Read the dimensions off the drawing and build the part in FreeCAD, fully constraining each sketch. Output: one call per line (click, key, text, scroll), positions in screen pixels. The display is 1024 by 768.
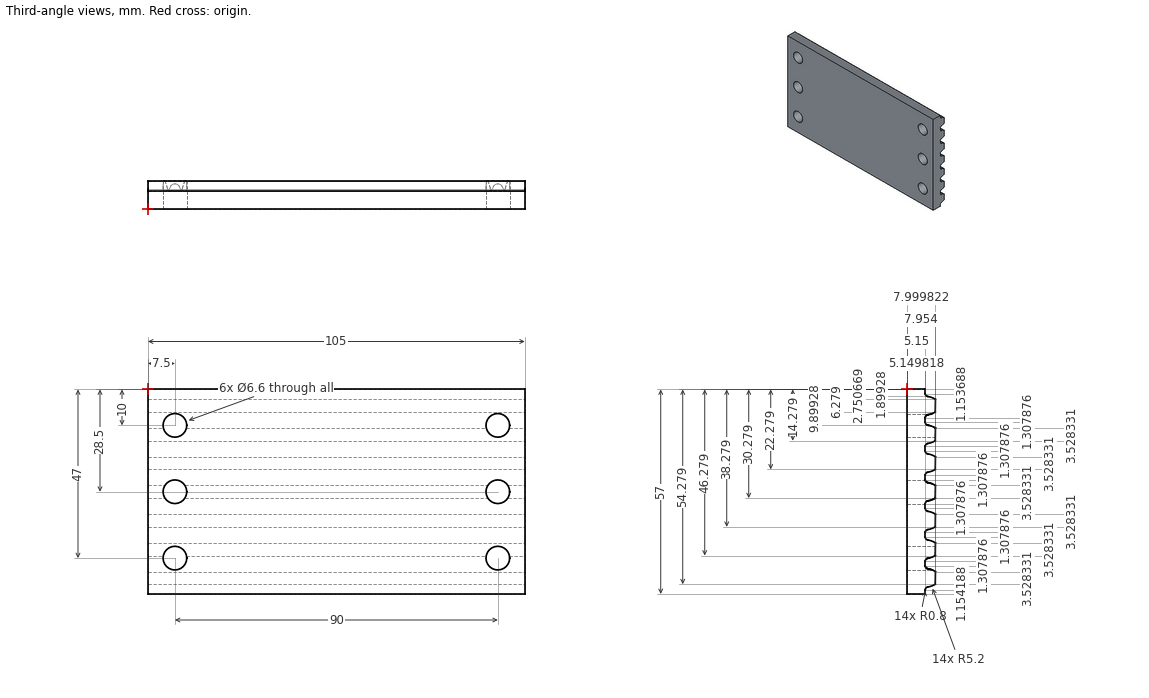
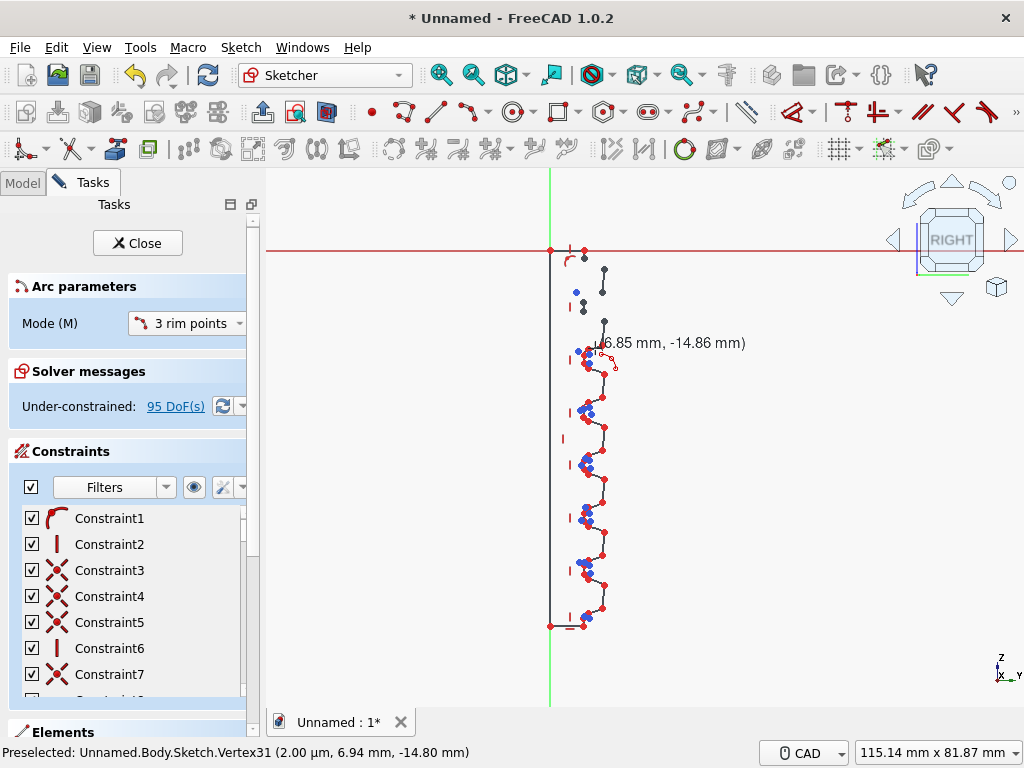
scroll(603, 321, up, 2)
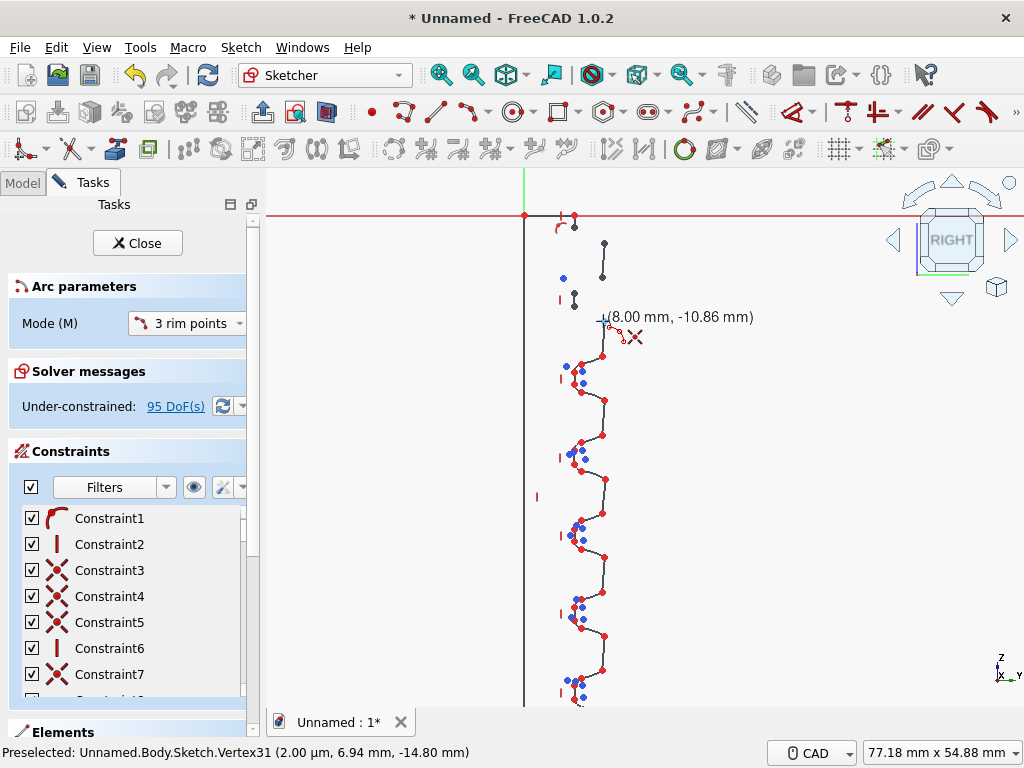
click(605, 322)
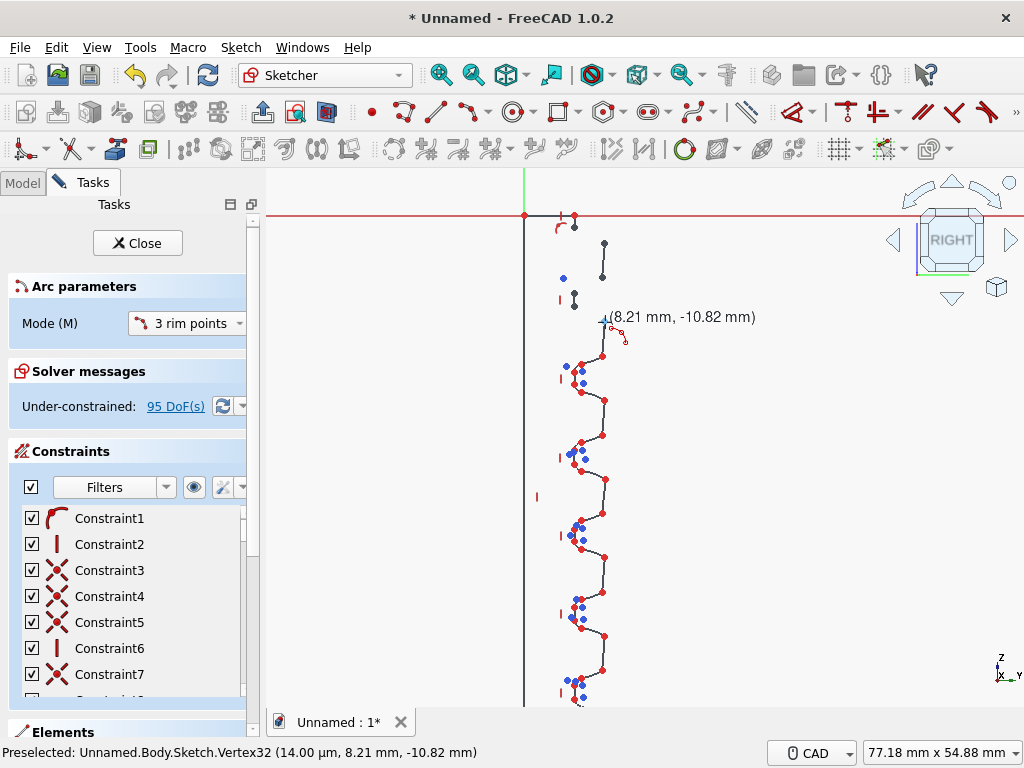
scroll(582, 313, up, 5)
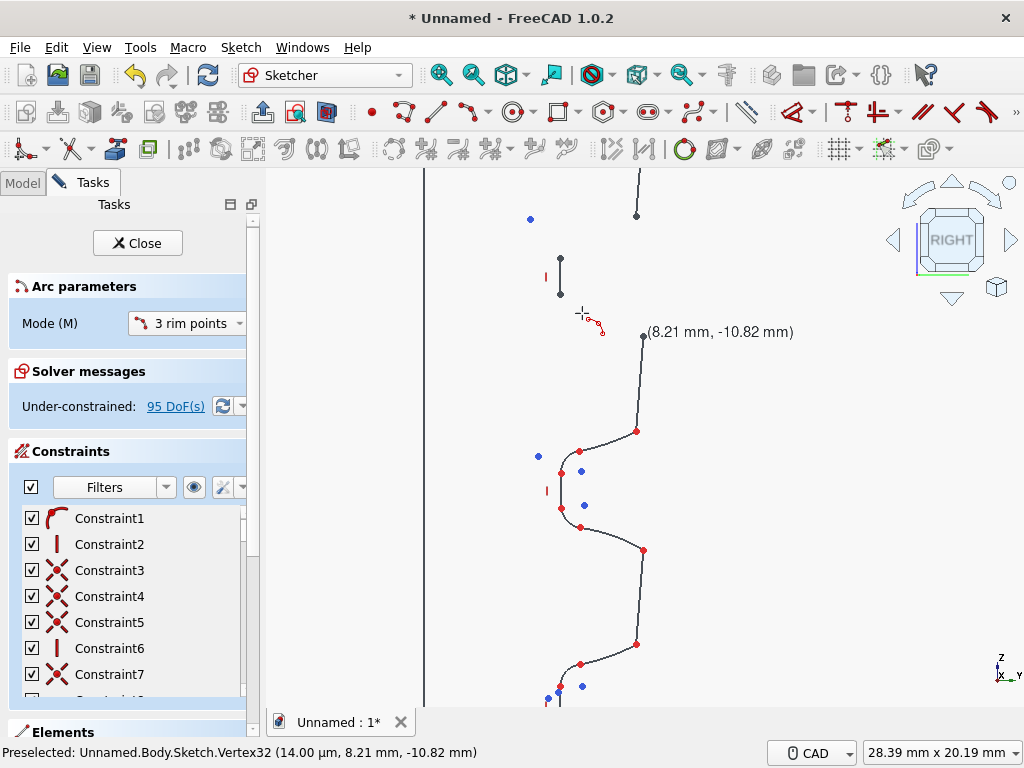
click(580, 314)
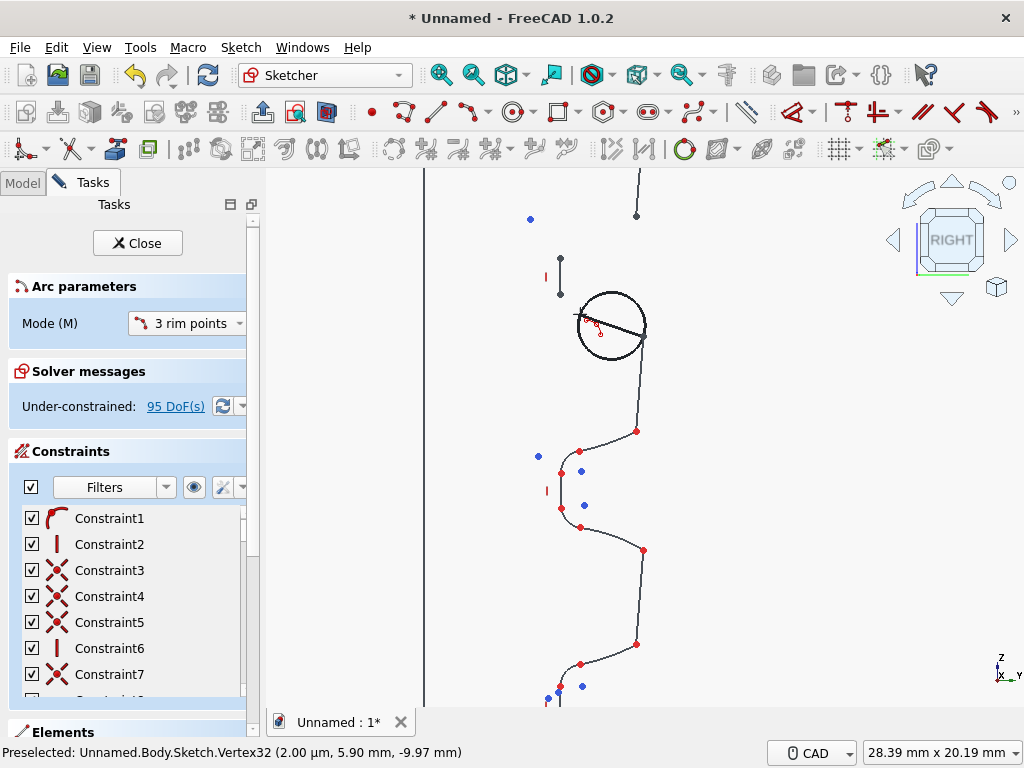
scroll(610, 321, up, 8)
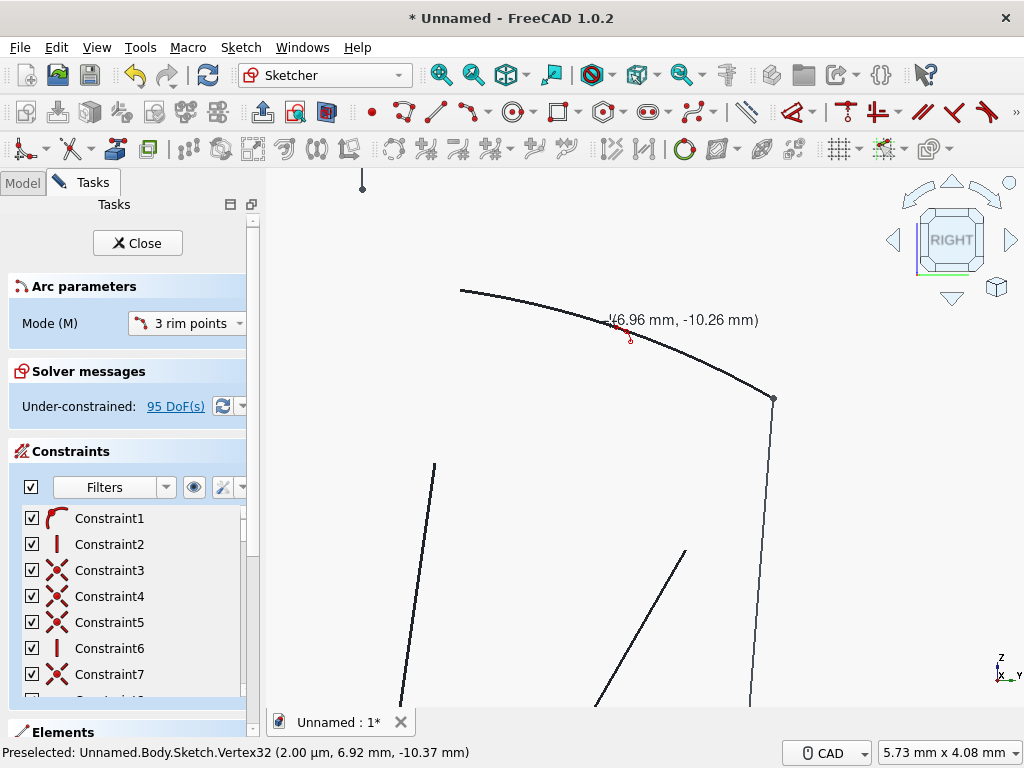
click(609, 321)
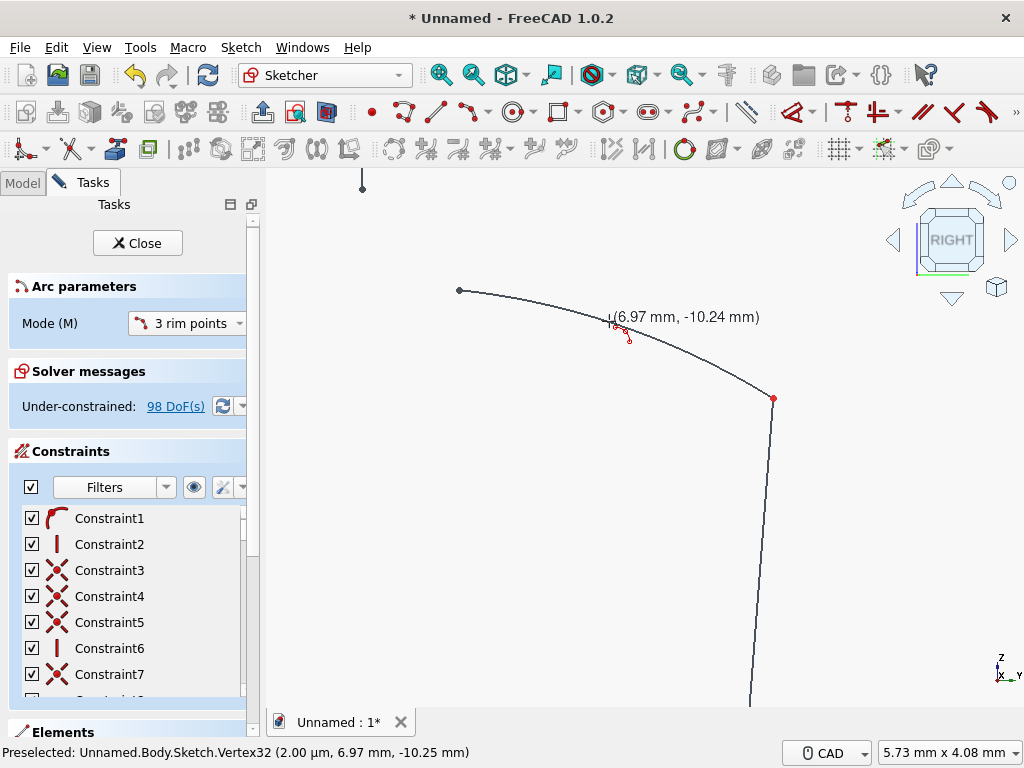
scroll(595, 317, down, 15)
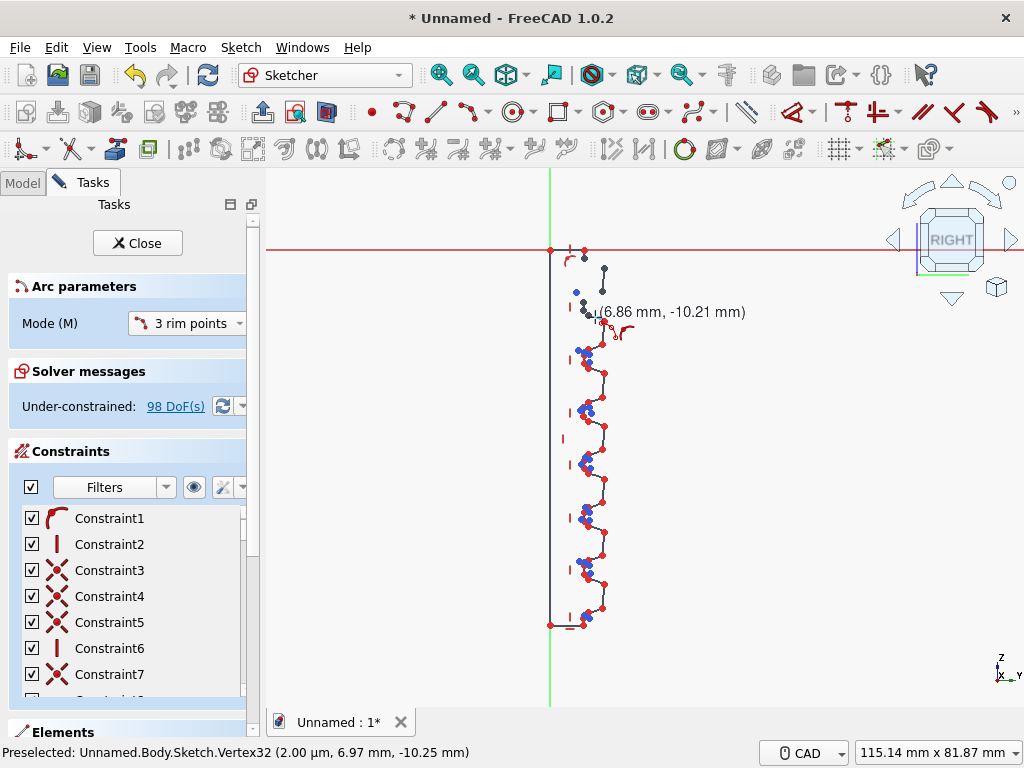
scroll(589, 316, up, 7)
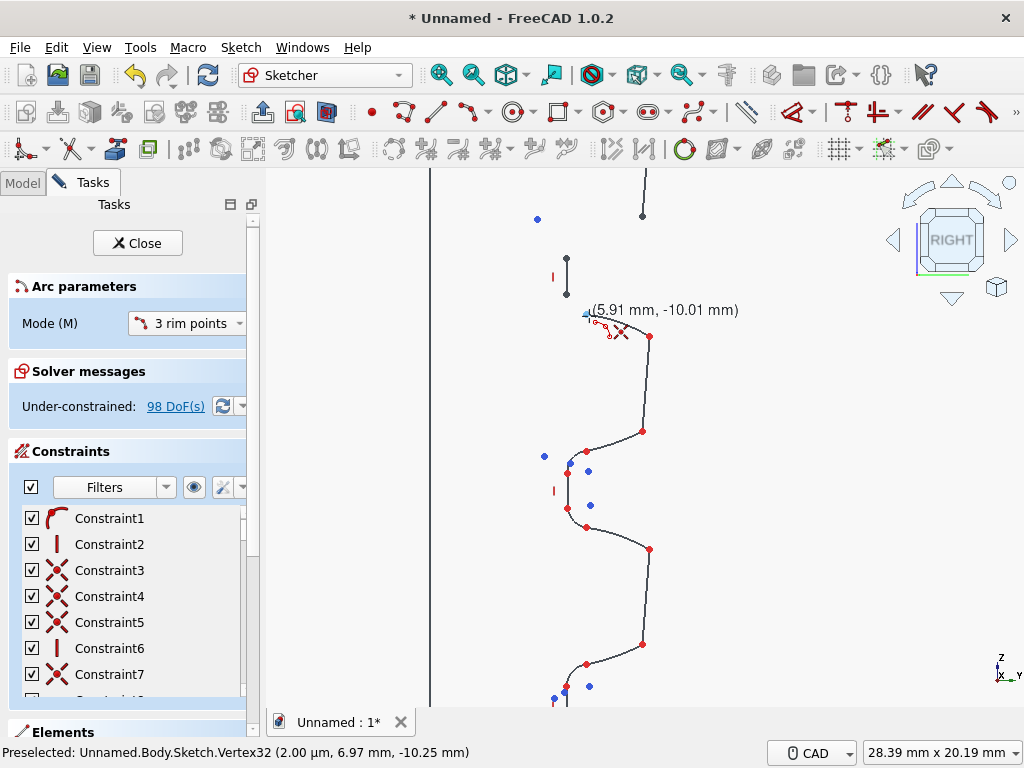
click(586, 315)
click(567, 294)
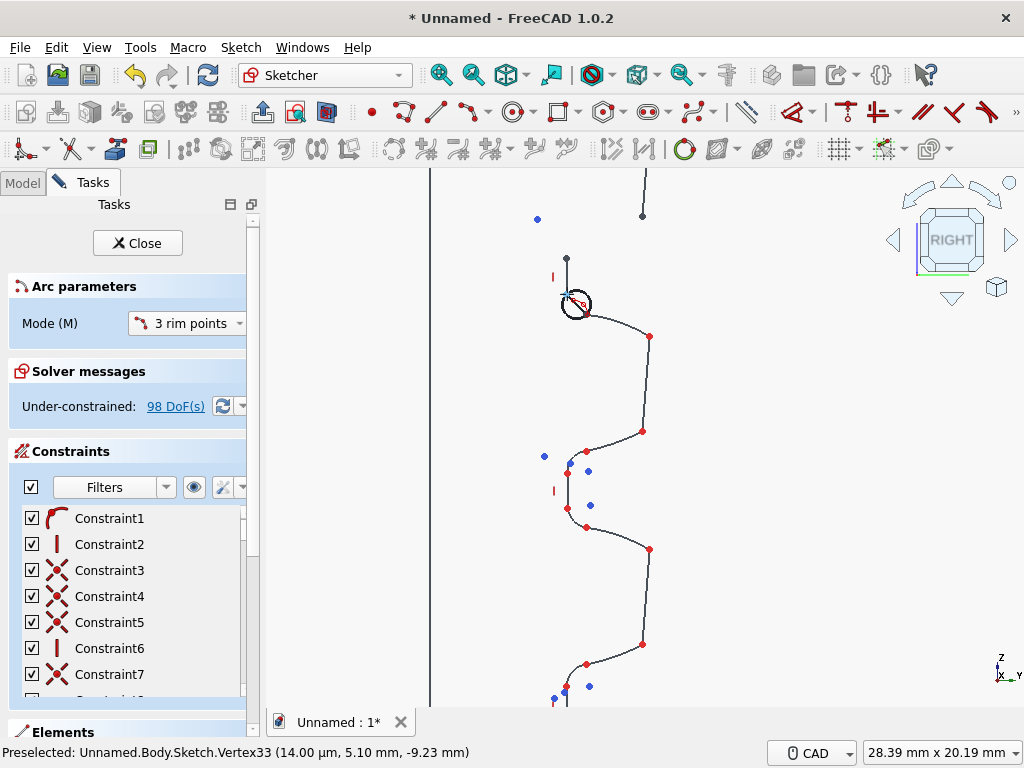
scroll(573, 306, up, 6)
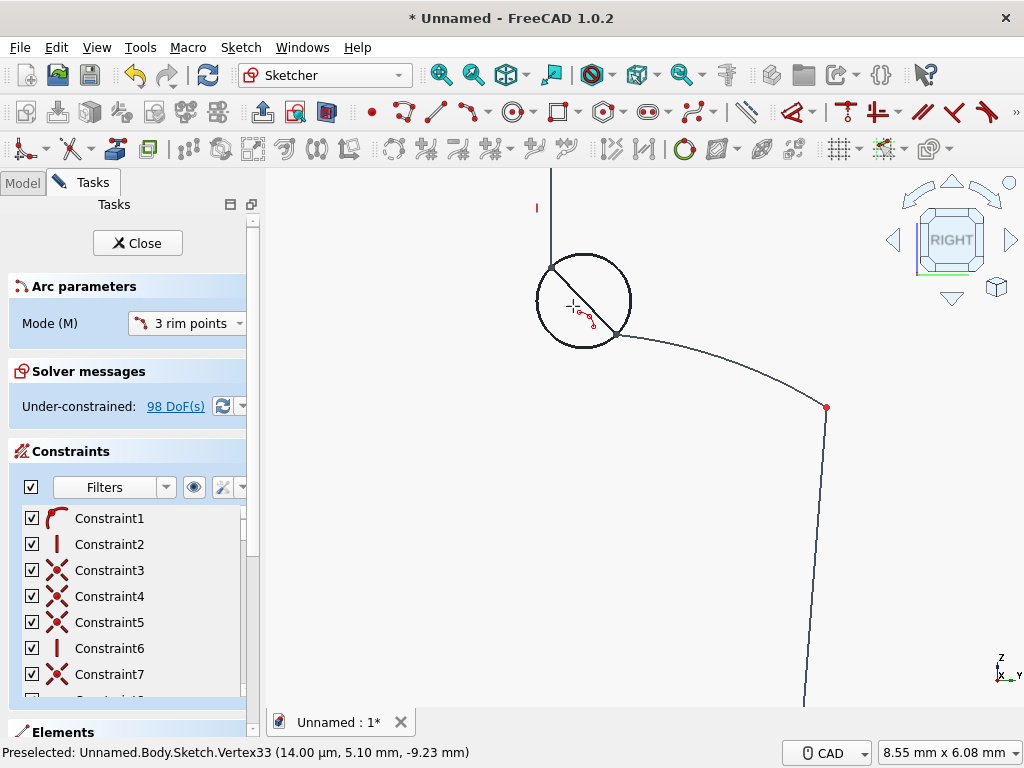
click(573, 307)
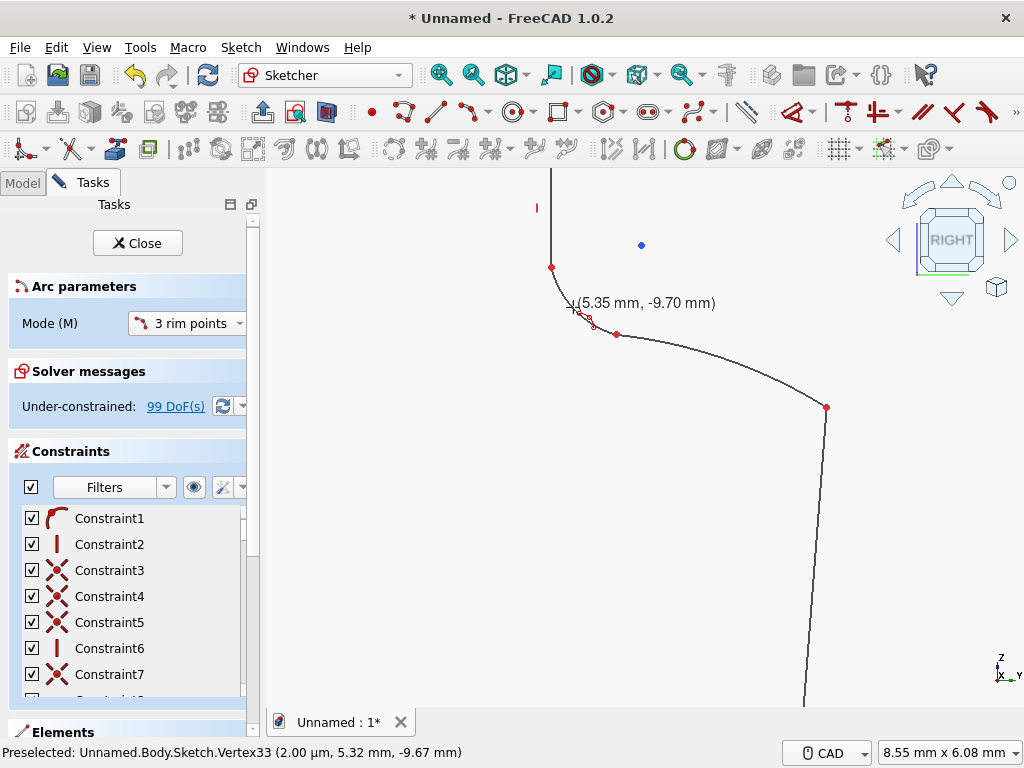
scroll(586, 314, down, 13)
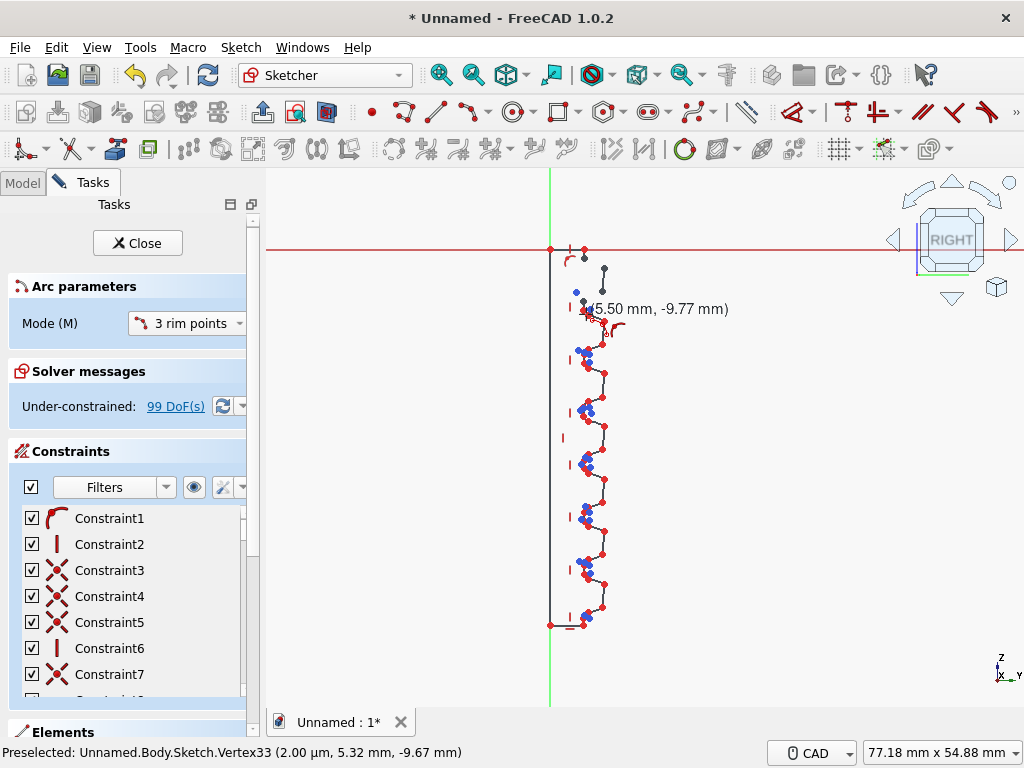
scroll(584, 302, up, 7)